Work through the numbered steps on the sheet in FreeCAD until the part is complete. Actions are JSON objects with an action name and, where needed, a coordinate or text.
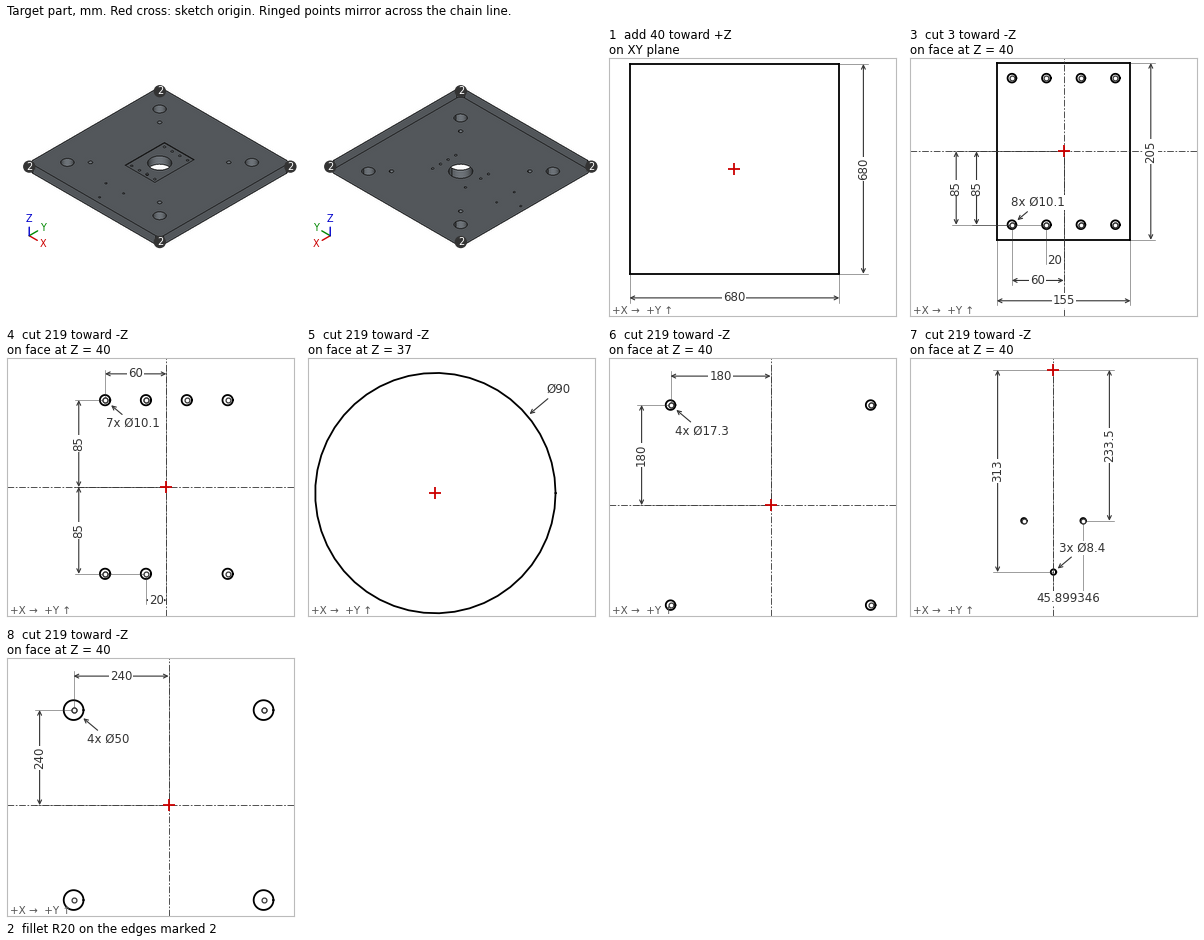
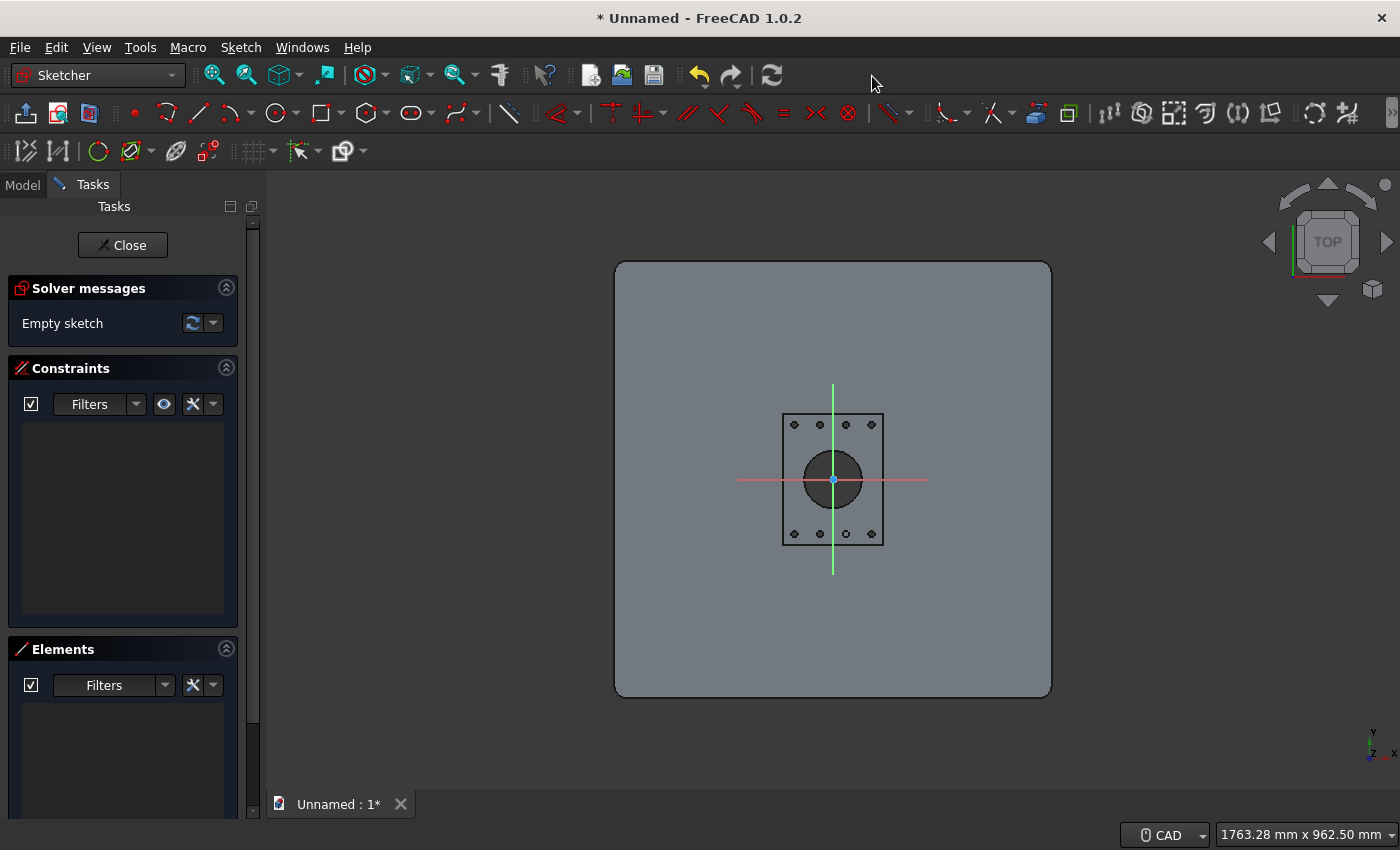
{"action": "scroll", "coordinate": [972, 479], "scroll_direction": "up", "scroll_amount": 2}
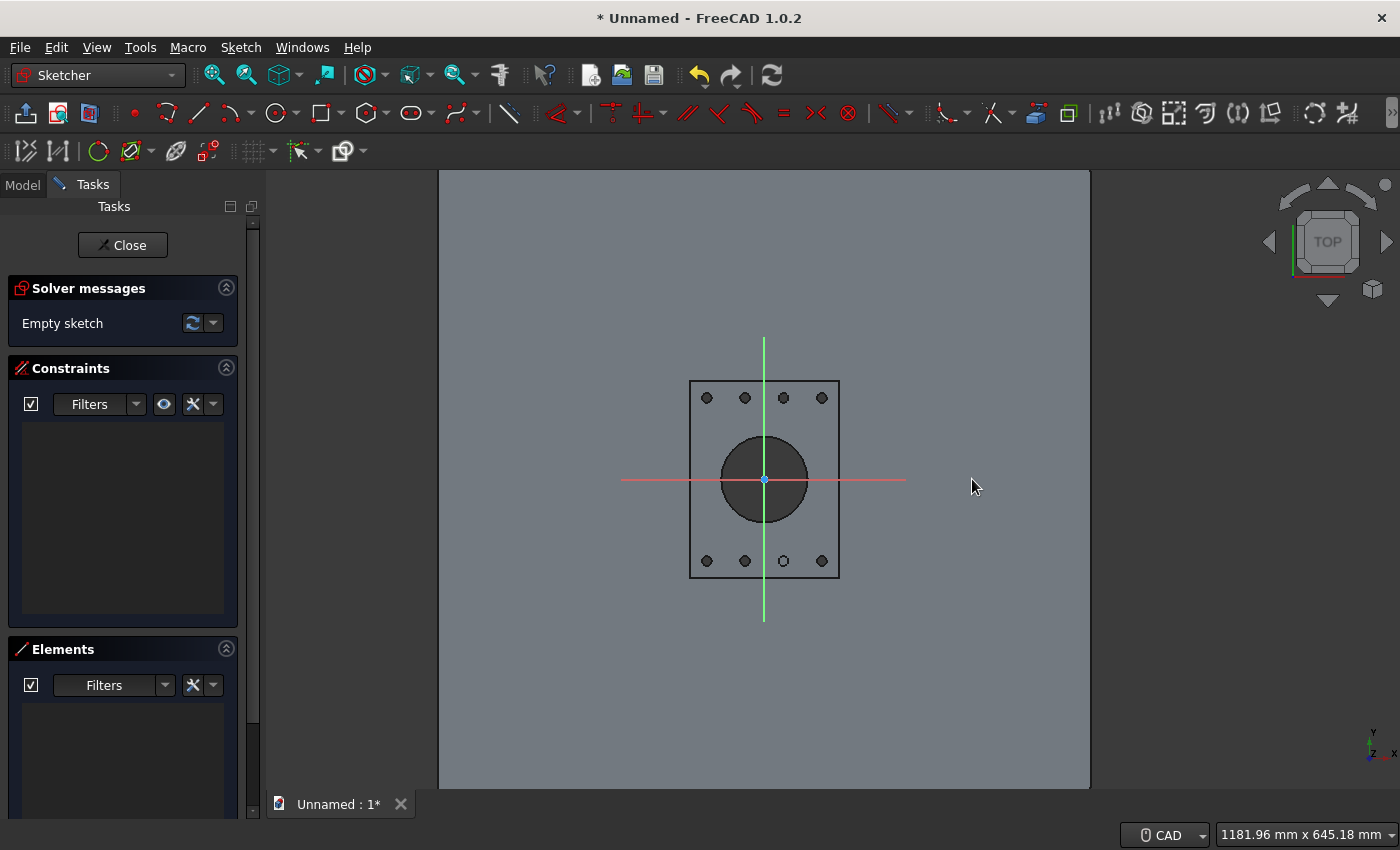
{"action": "left_click", "coordinate": [276, 114]}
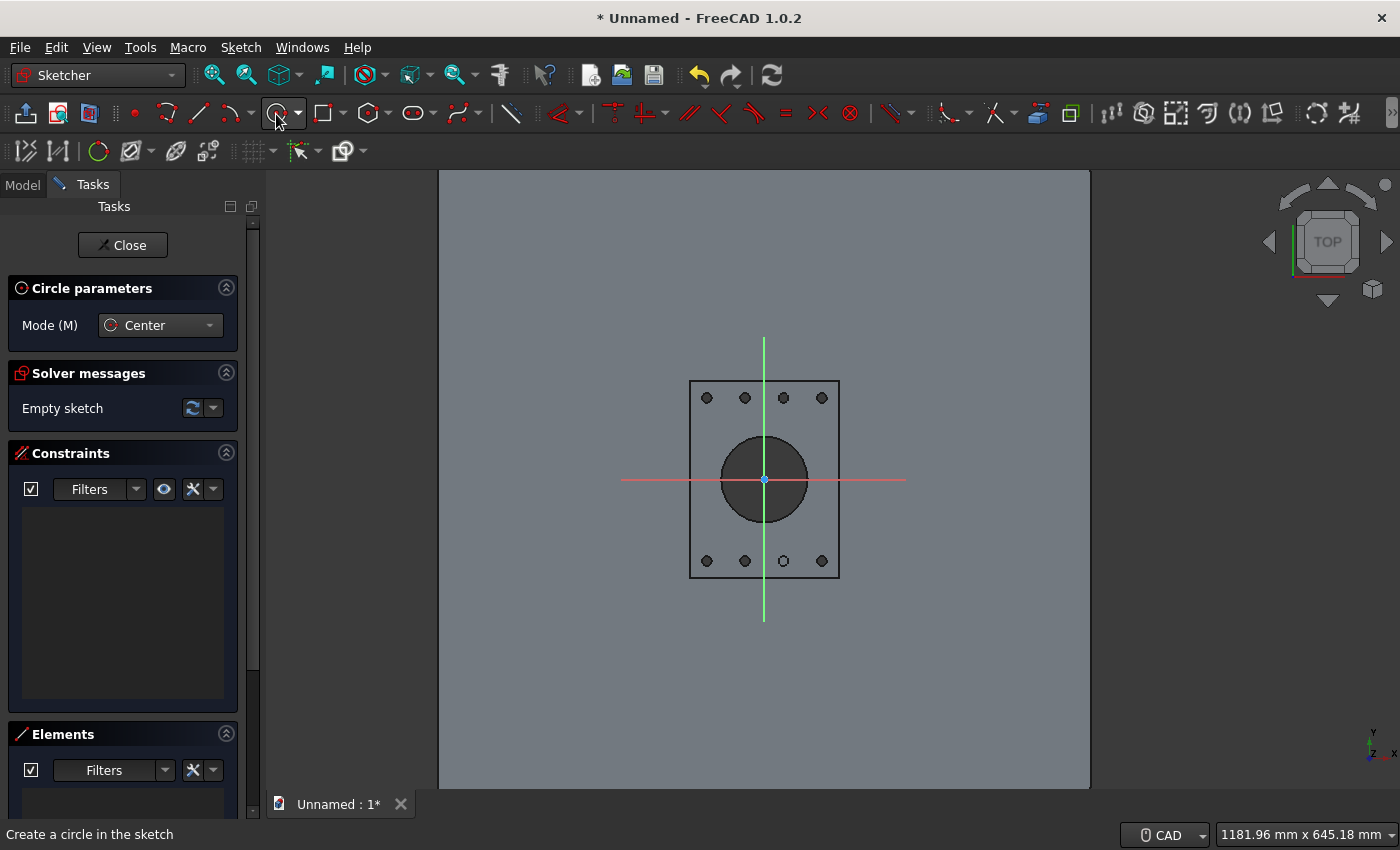
{"action": "scroll", "coordinate": [592, 307], "scroll_direction": "up", "scroll_amount": 6}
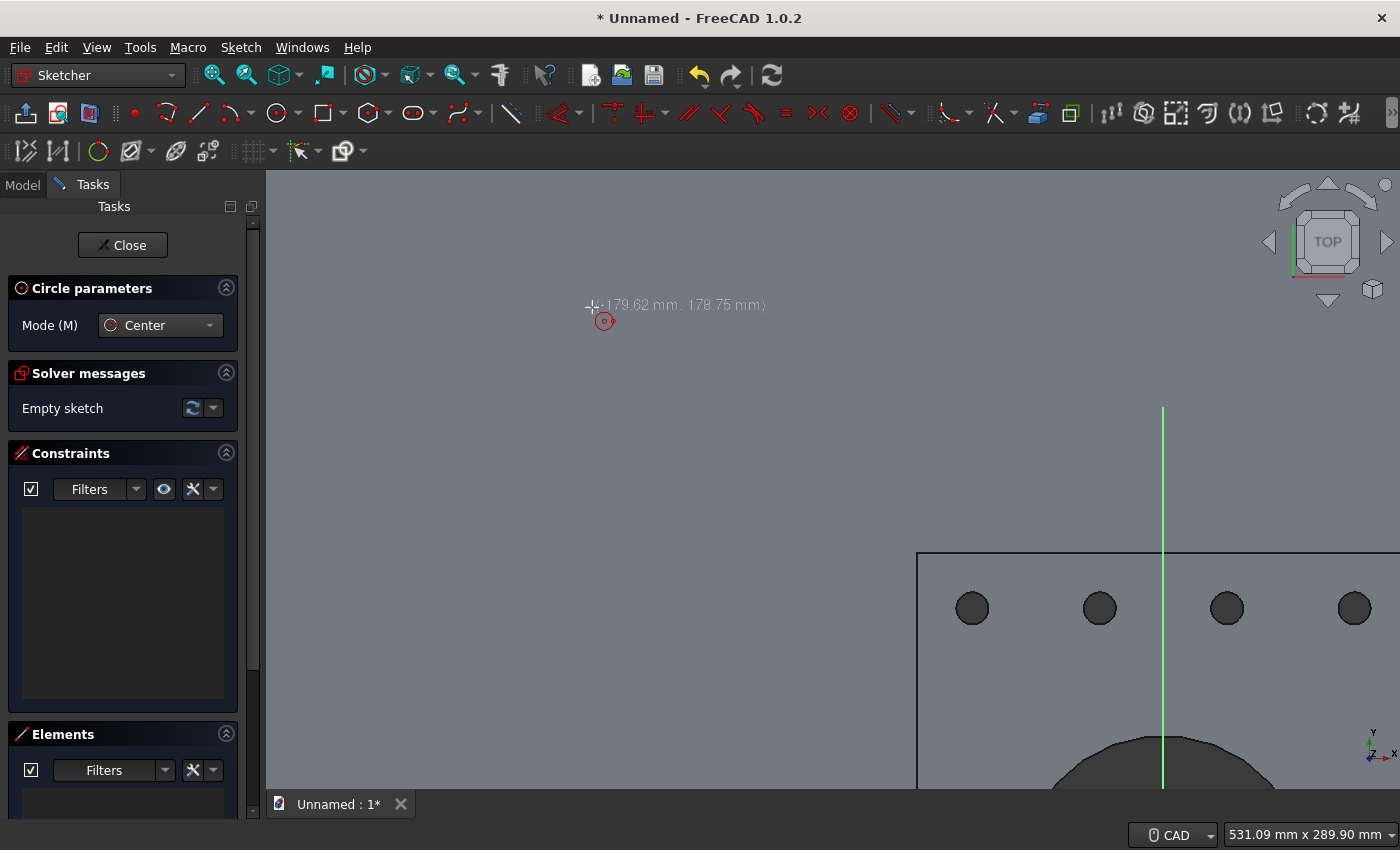
{"action": "left_click", "coordinate": [590, 306]}
{"action": "left_click", "coordinate": [610, 286]}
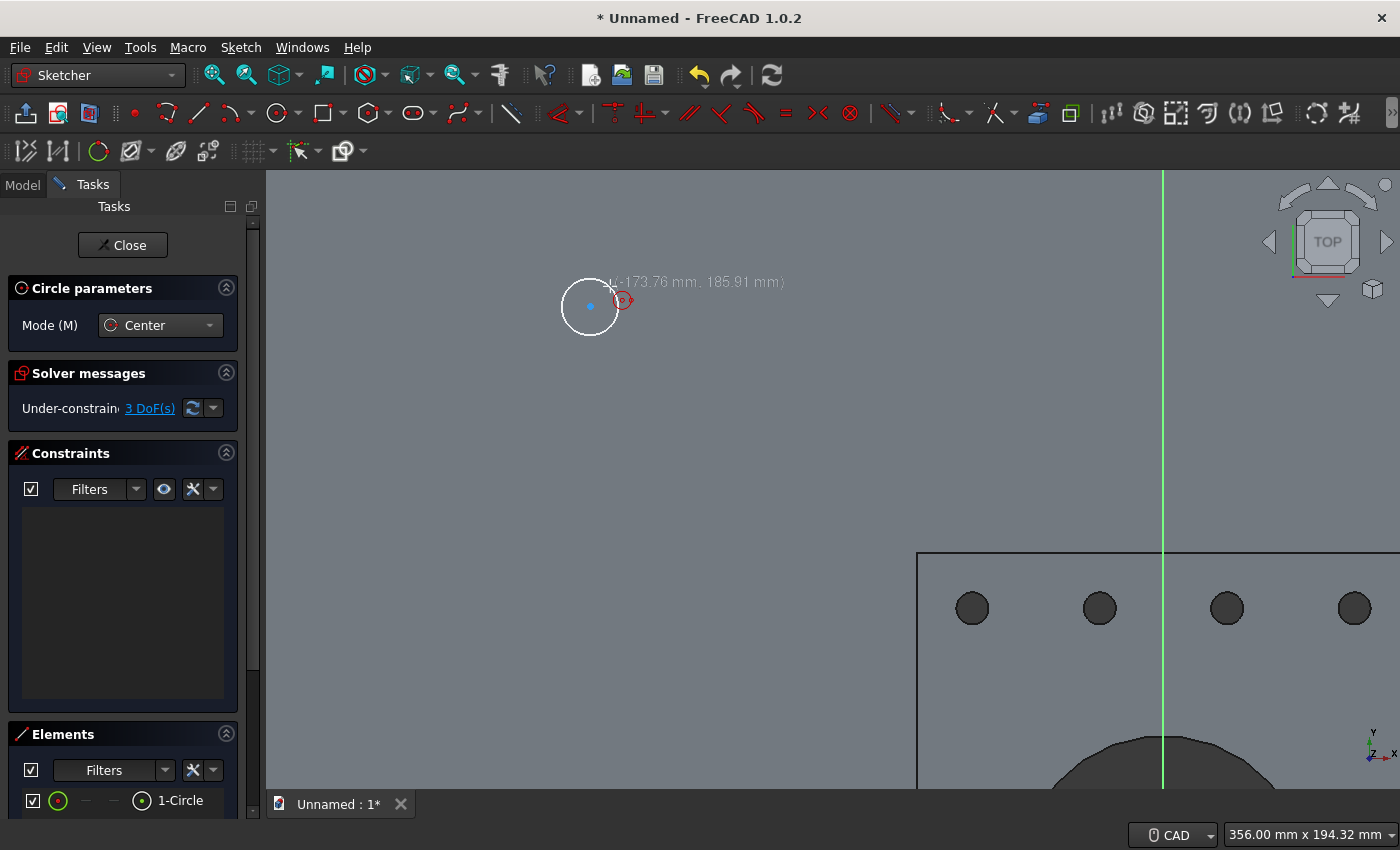
{"action": "scroll", "coordinate": [593, 307], "scroll_direction": "down", "scroll_amount": 6}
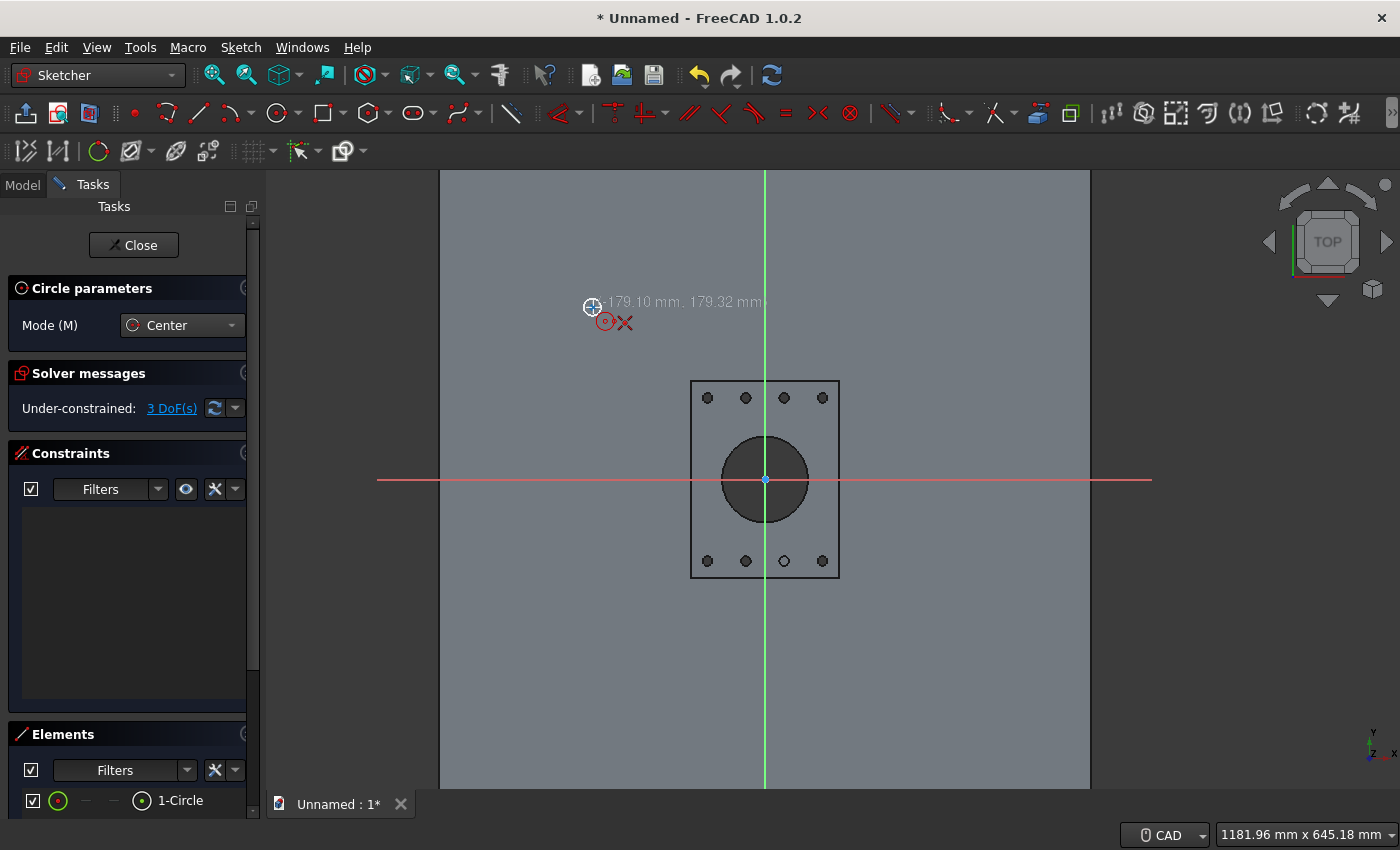
{"action": "scroll", "coordinate": [938, 307], "scroll_direction": "up", "scroll_amount": 6}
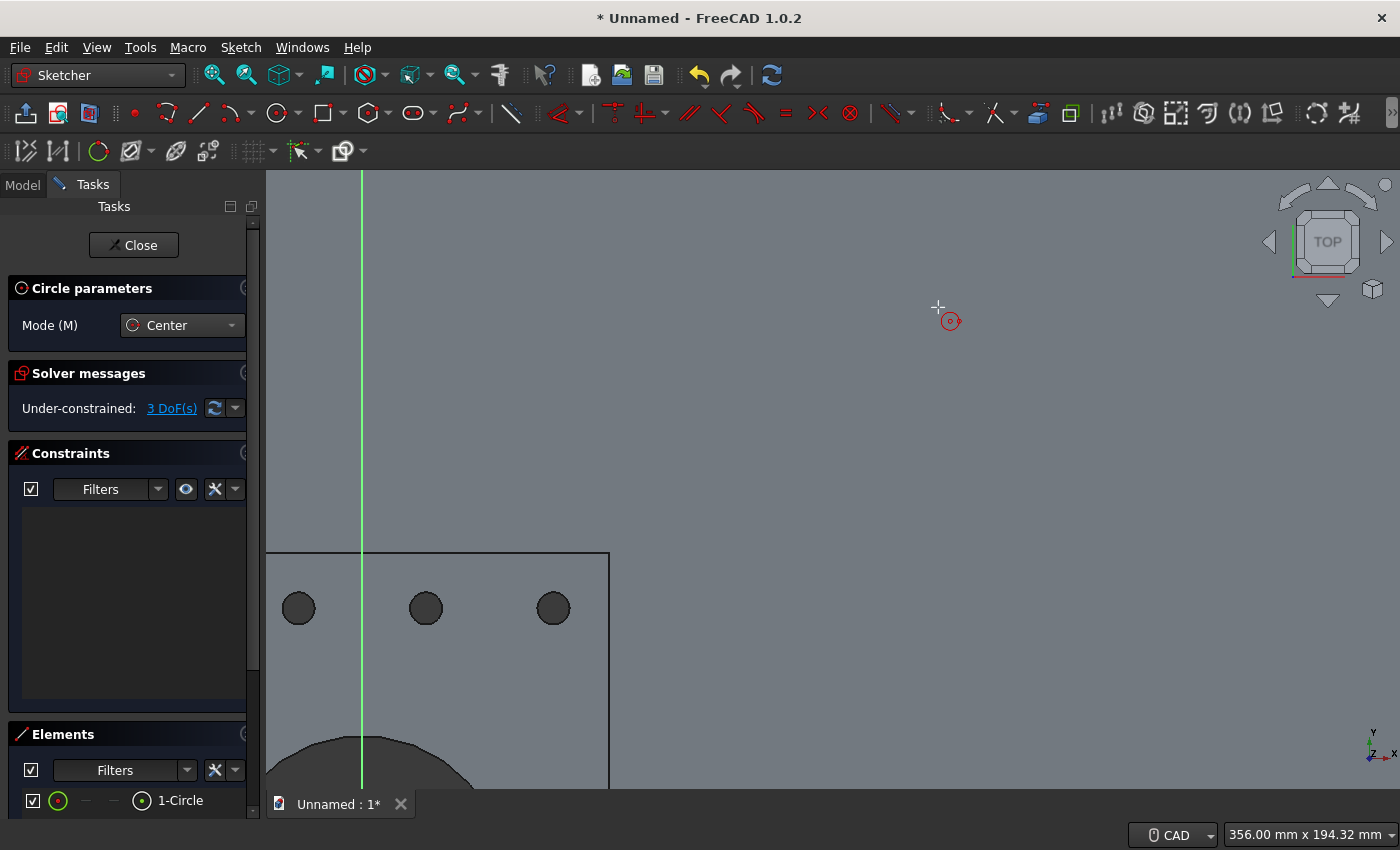
{"action": "left_click", "coordinate": [936, 306]}
{"action": "left_click", "coordinate": [955, 286]}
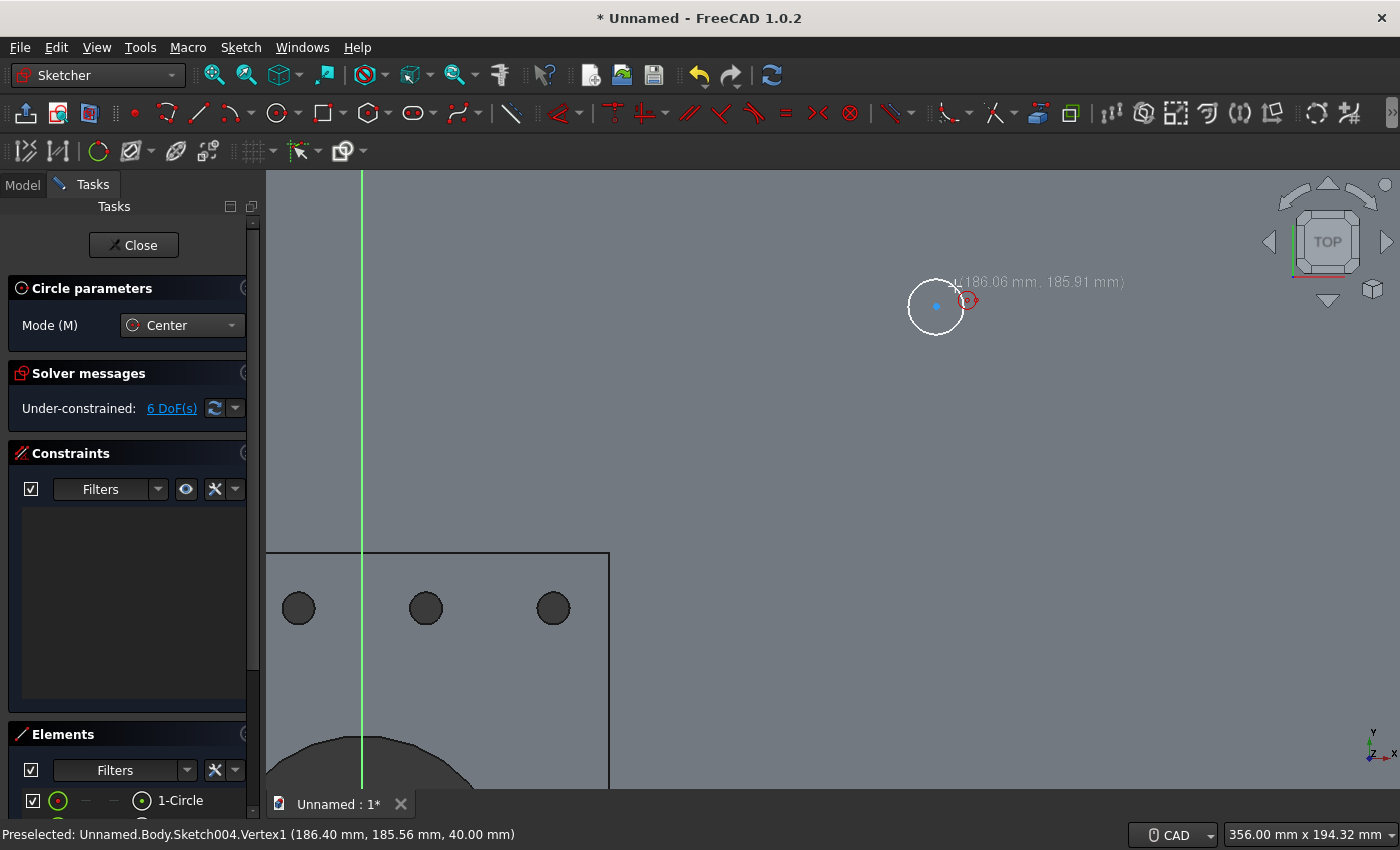
{"action": "scroll", "coordinate": [938, 307], "scroll_direction": "down", "scroll_amount": 6}